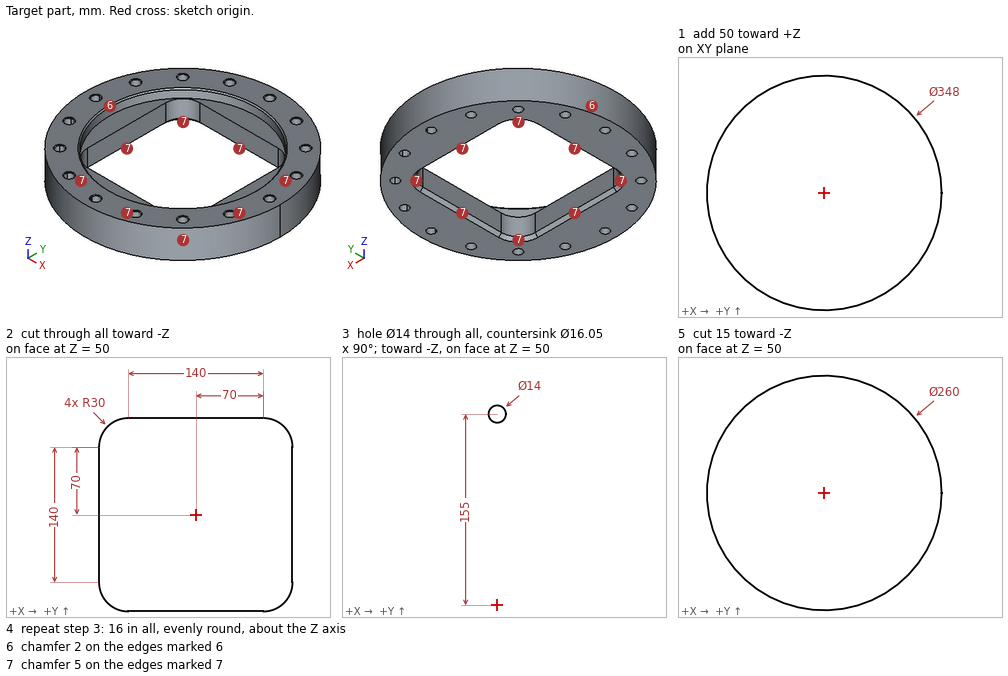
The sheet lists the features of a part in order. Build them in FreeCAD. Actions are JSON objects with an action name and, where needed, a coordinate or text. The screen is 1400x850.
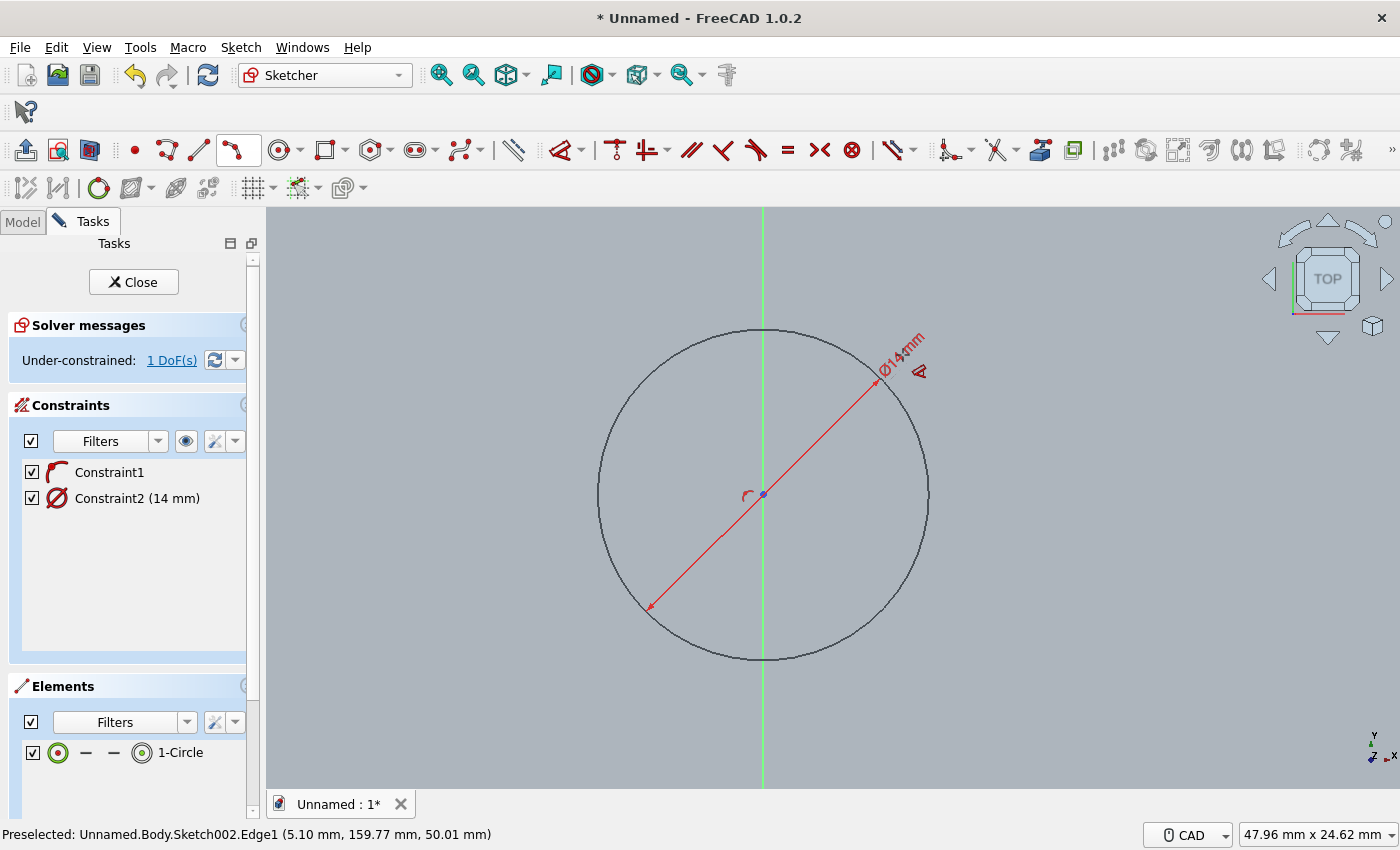
{"action": "left_click", "coordinate": [763, 495]}
{"action": "left_click", "coordinate": [797, 628]}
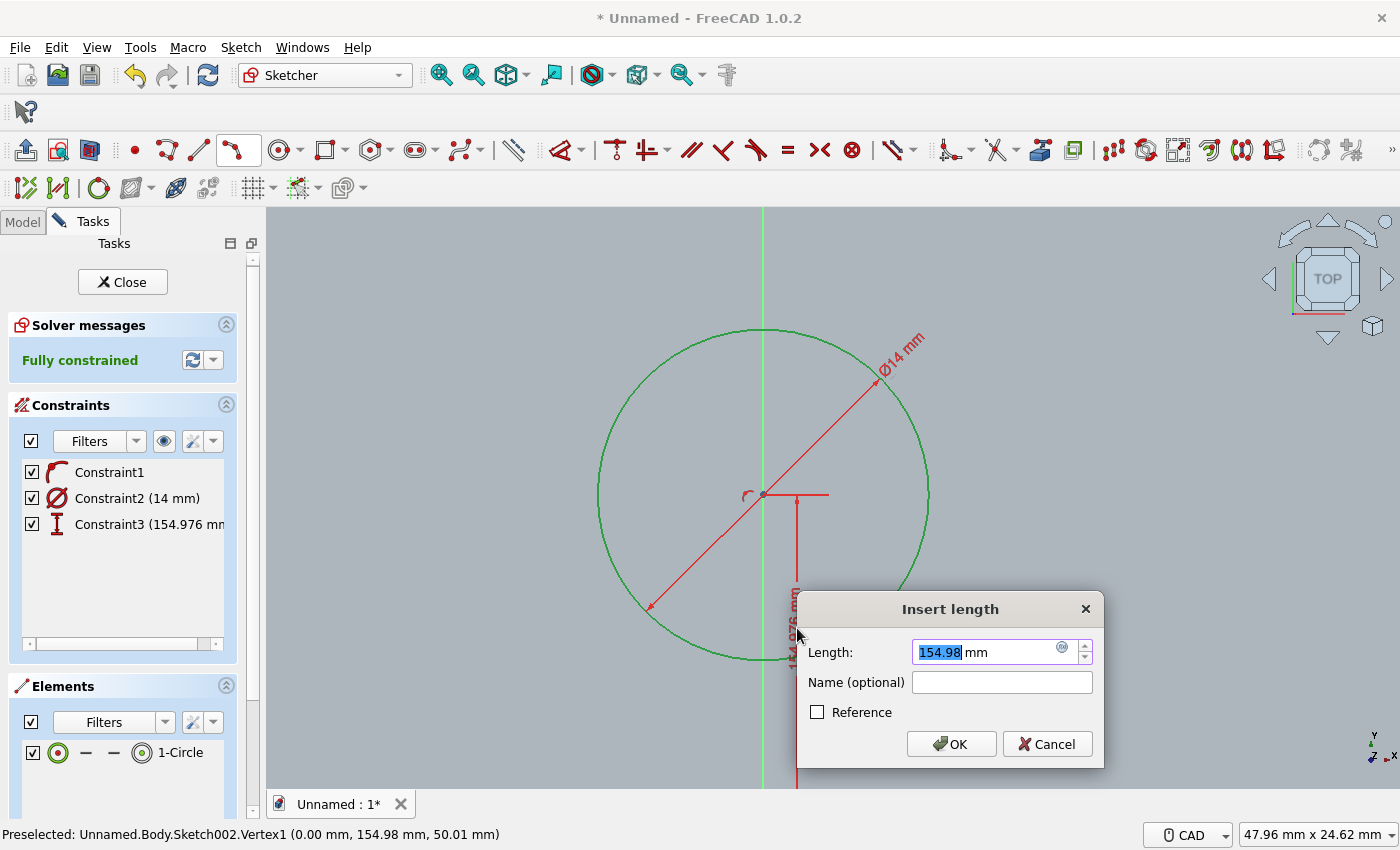
{"action": "type", "text": "155"}
{"action": "key", "text": "Return"}
{"action": "key", "text": "Escape"}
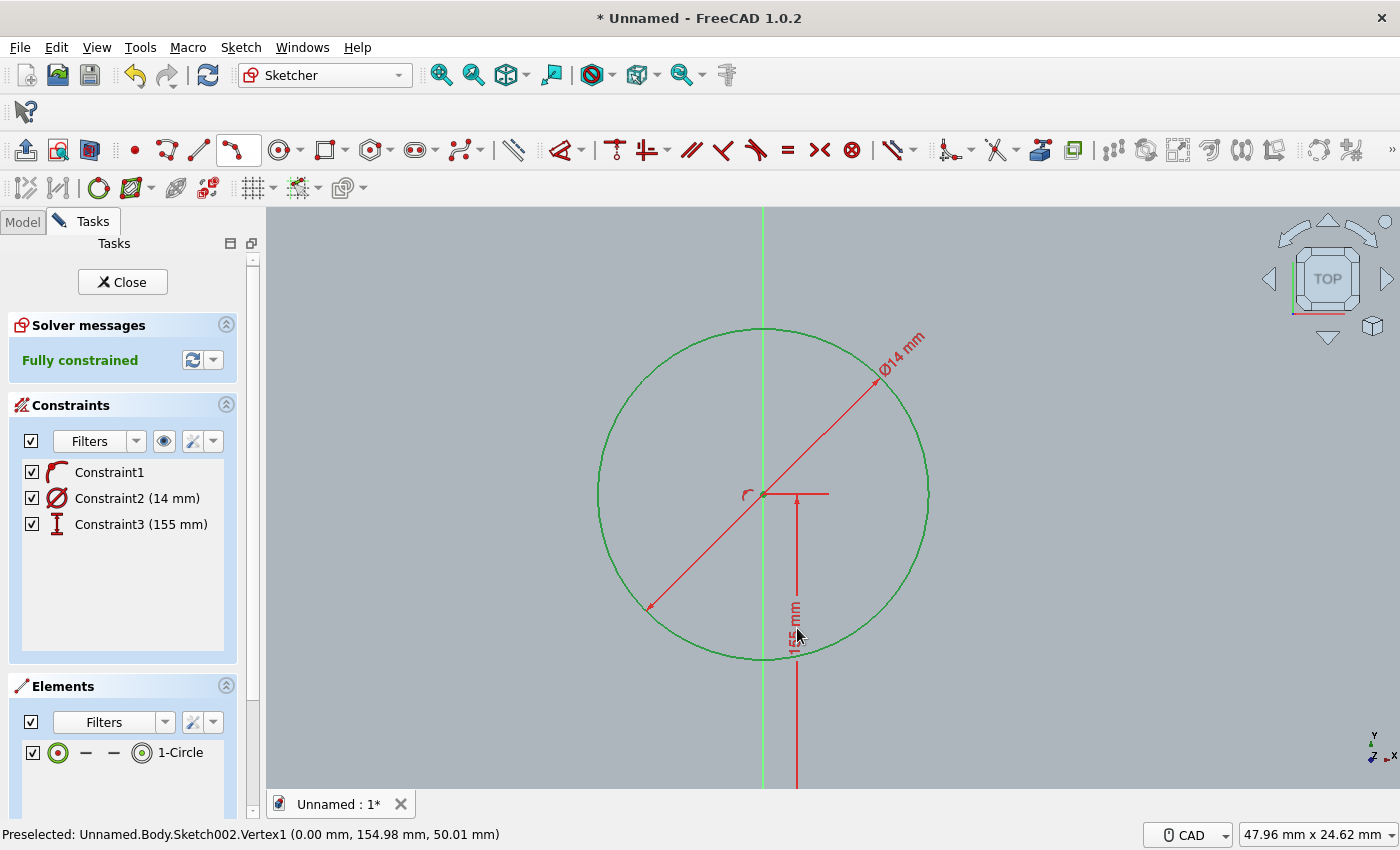
{"action": "left_click", "coordinate": [123, 282]}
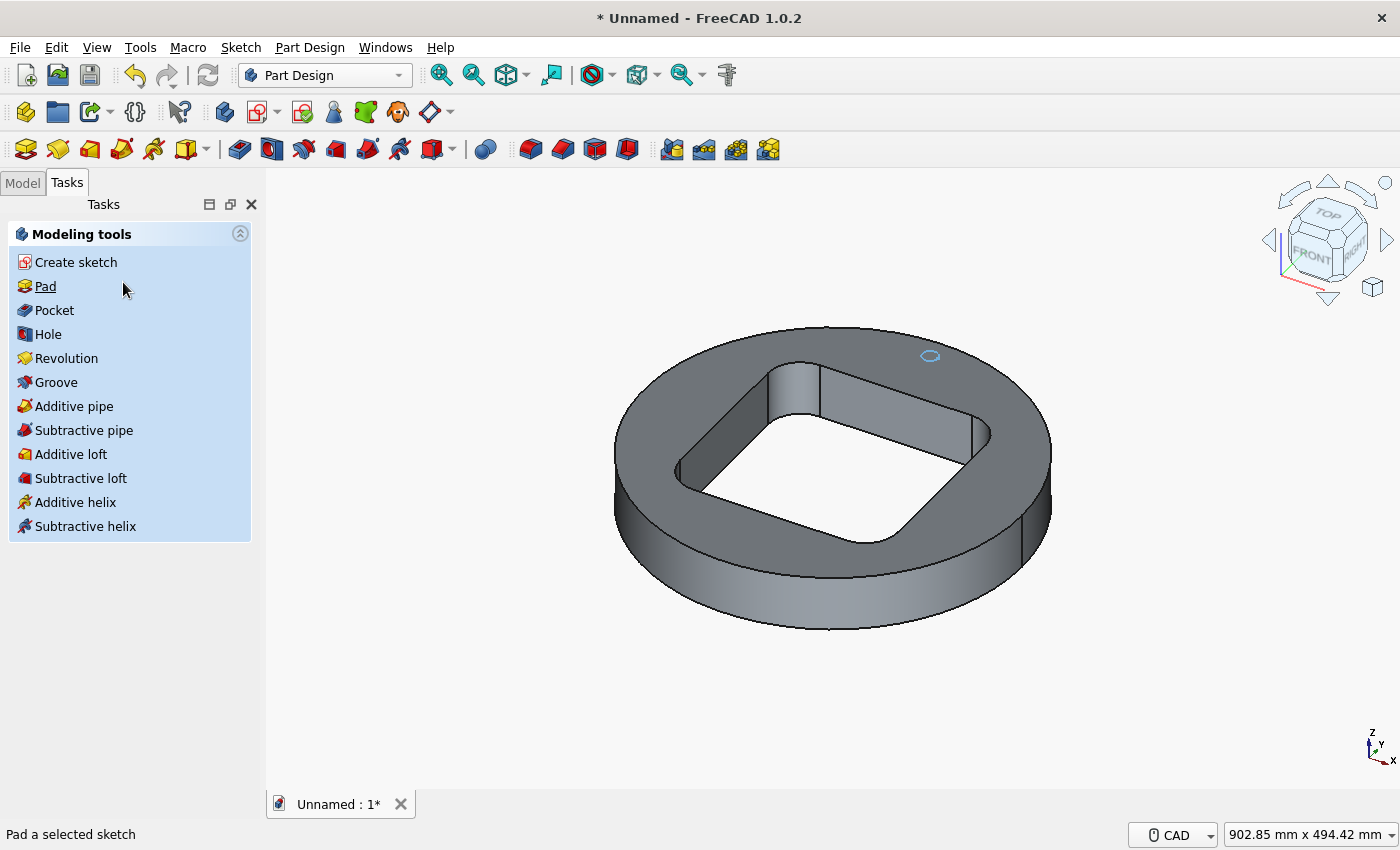
{"action": "left_click", "coordinate": [272, 150]}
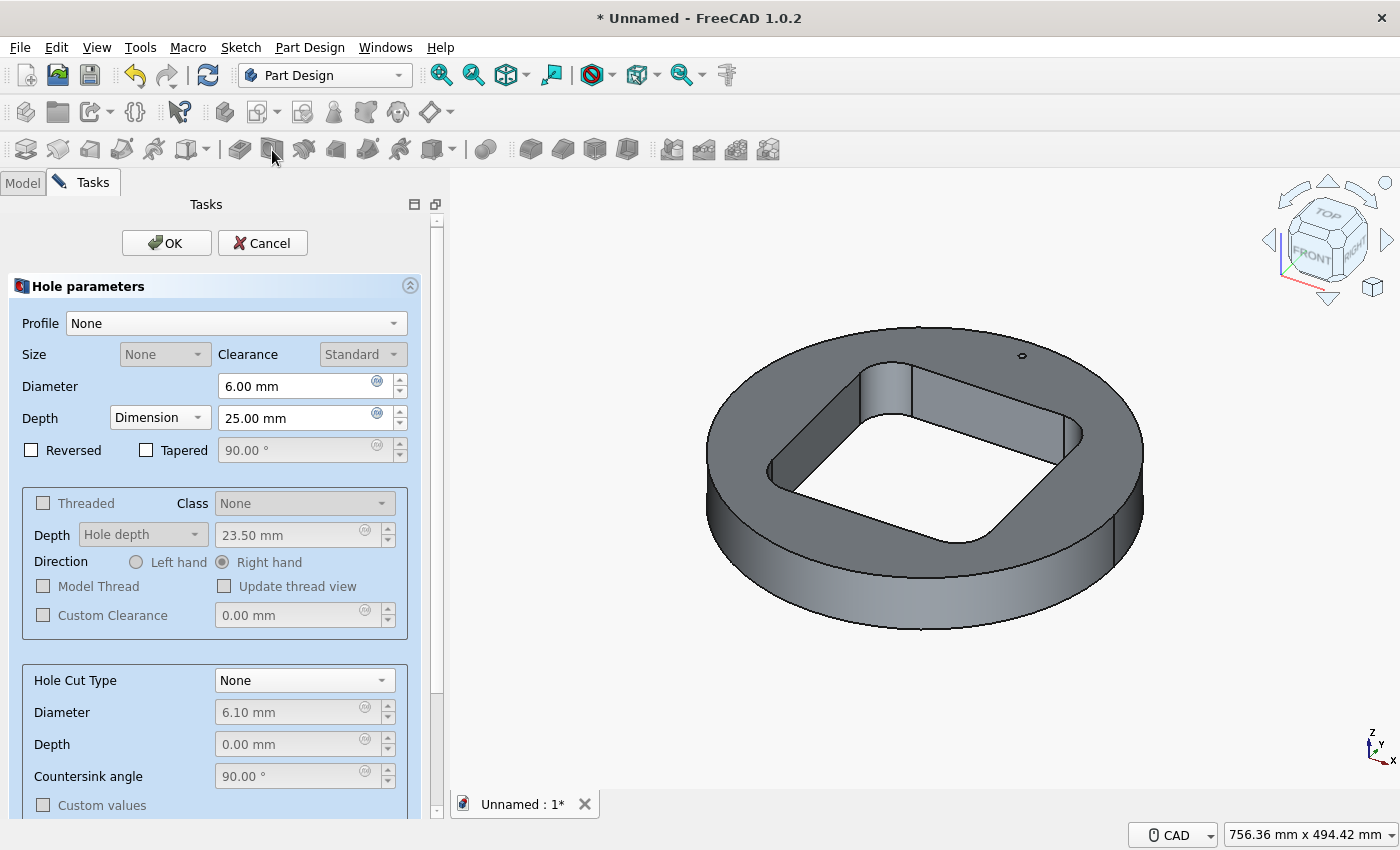
{"action": "triple_click", "coordinate": [305, 386]}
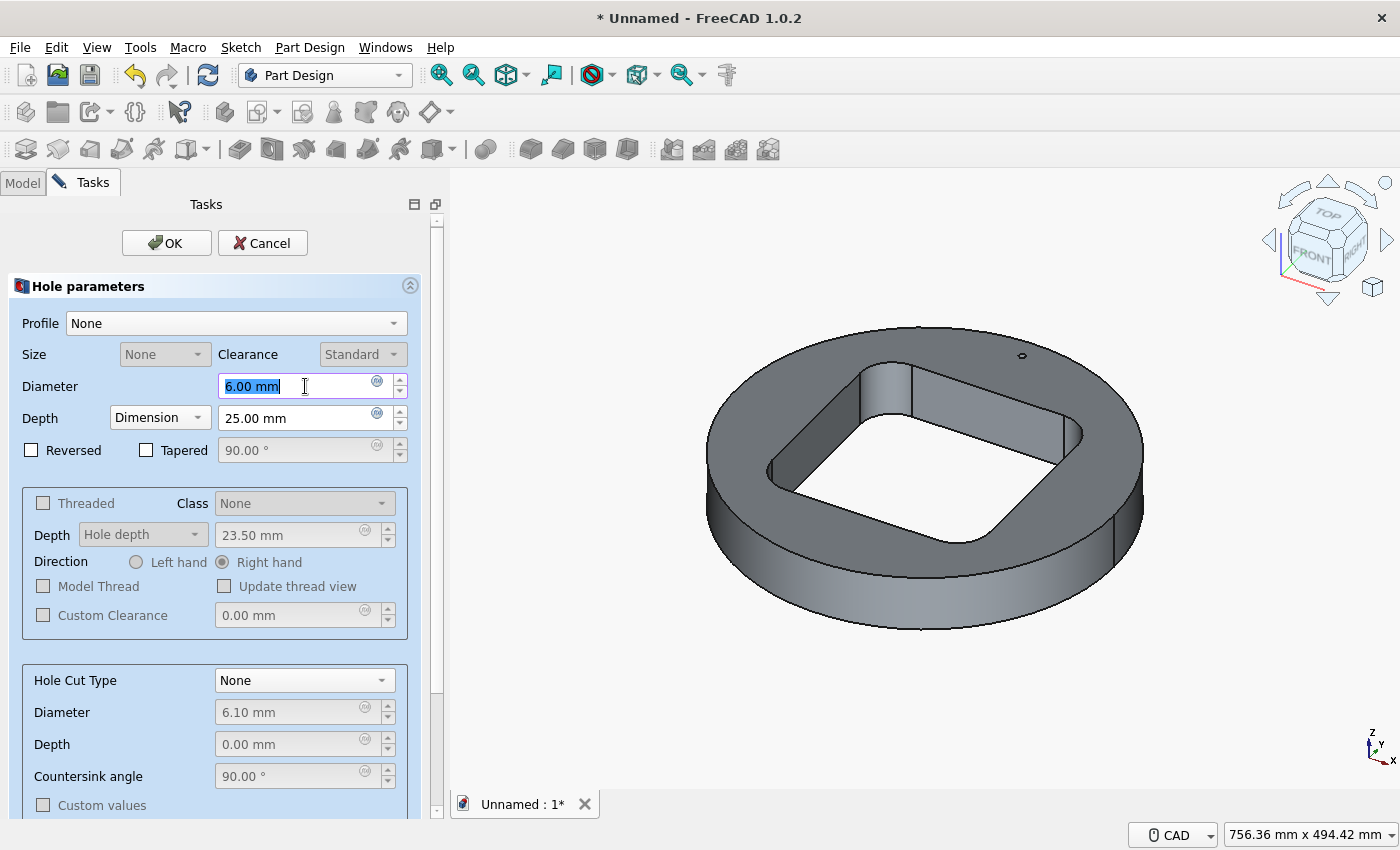
{"action": "type", "text": "14"}
{"action": "key", "text": "Tab"}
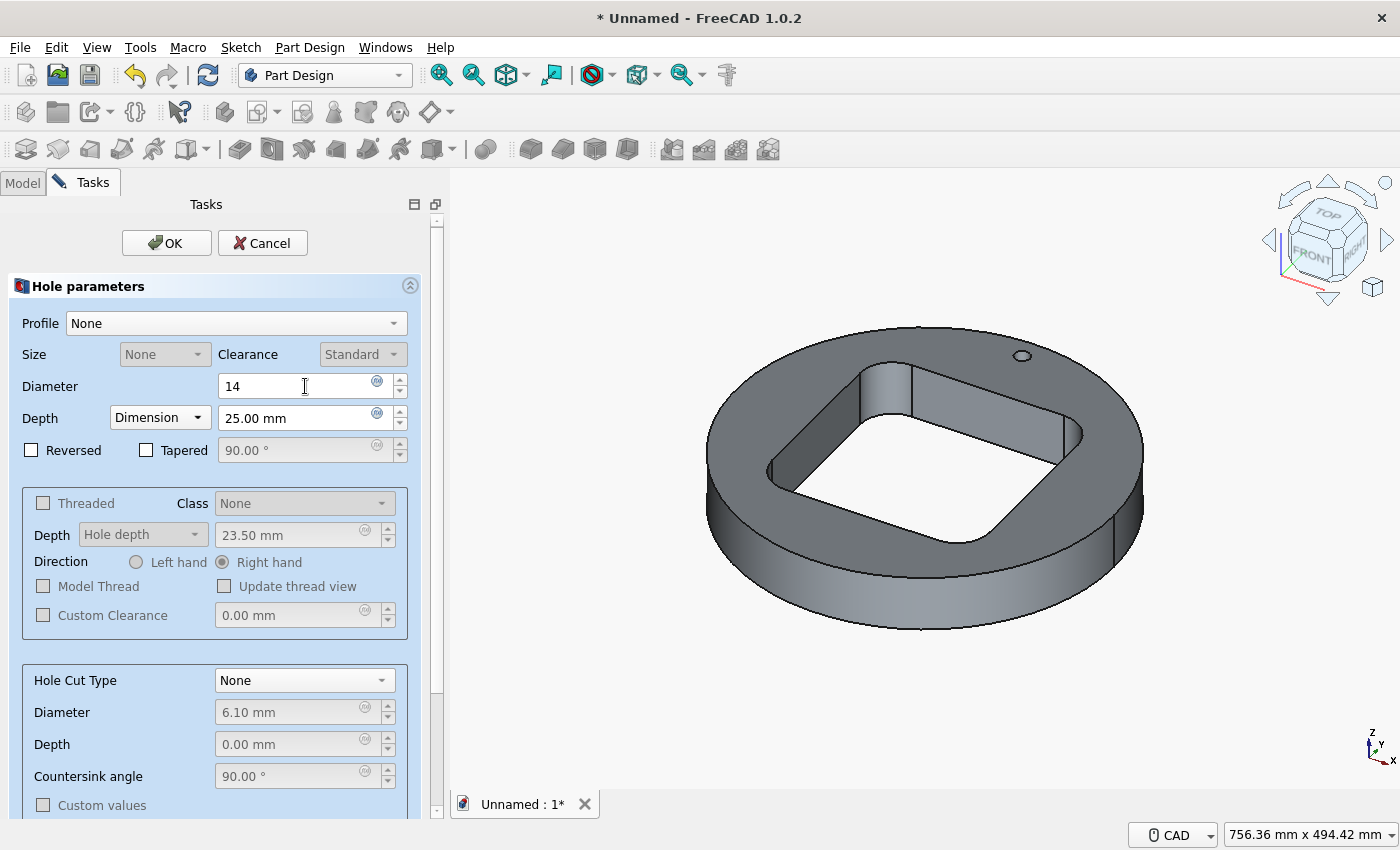
{"action": "left_click", "coordinate": [161, 418]}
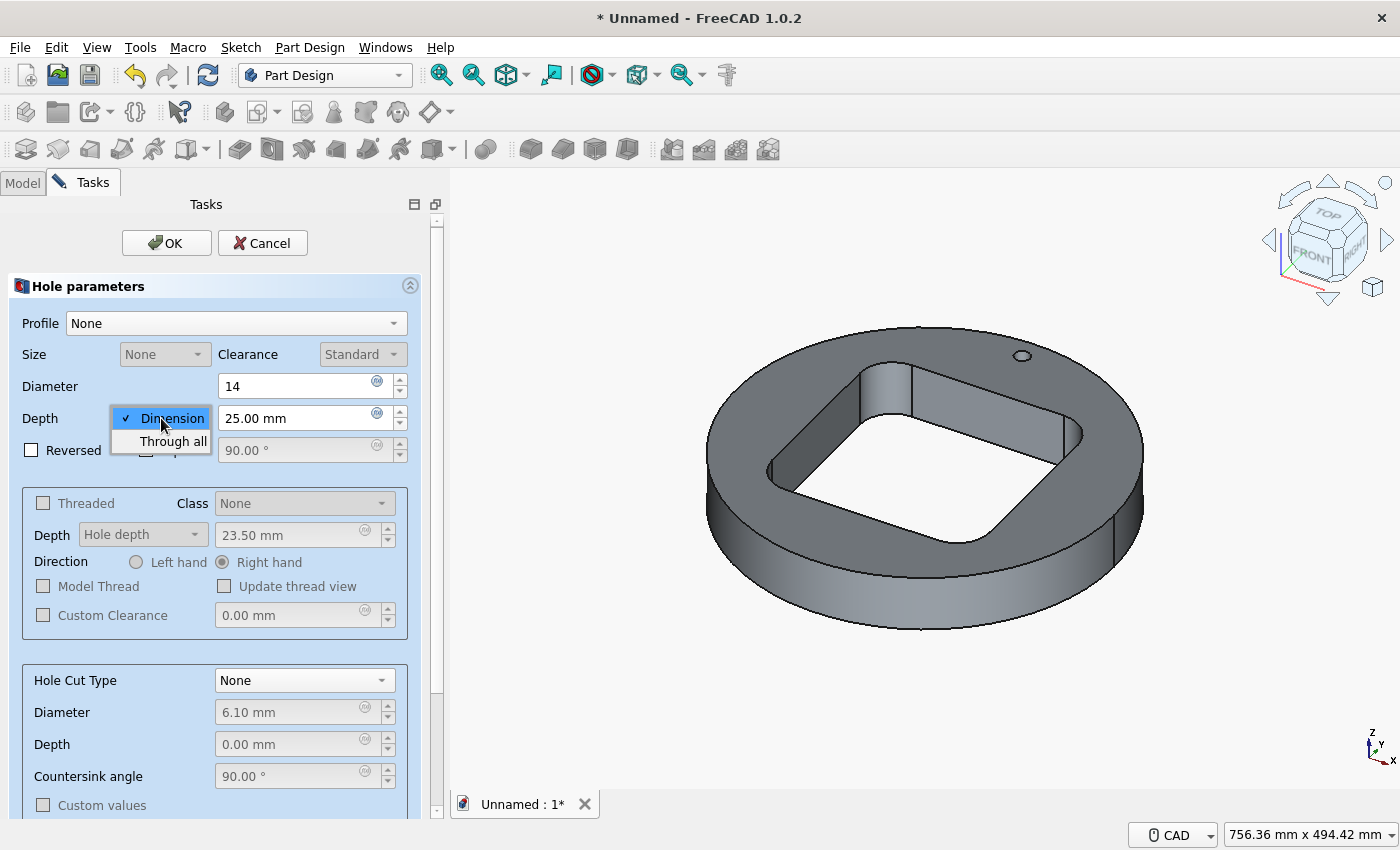
{"action": "left_click", "coordinate": [160, 442]}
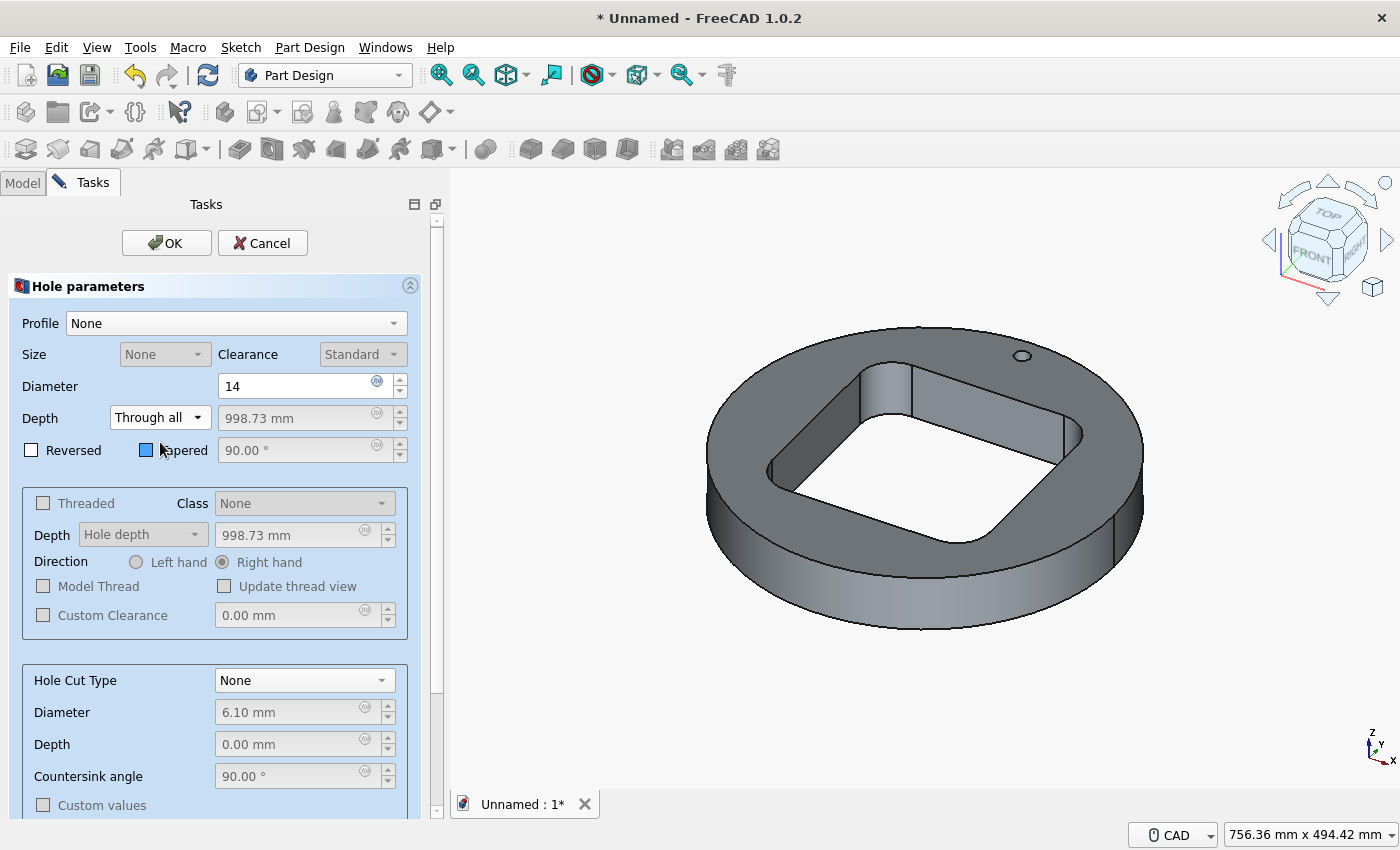
{"action": "left_click", "coordinate": [306, 680]}